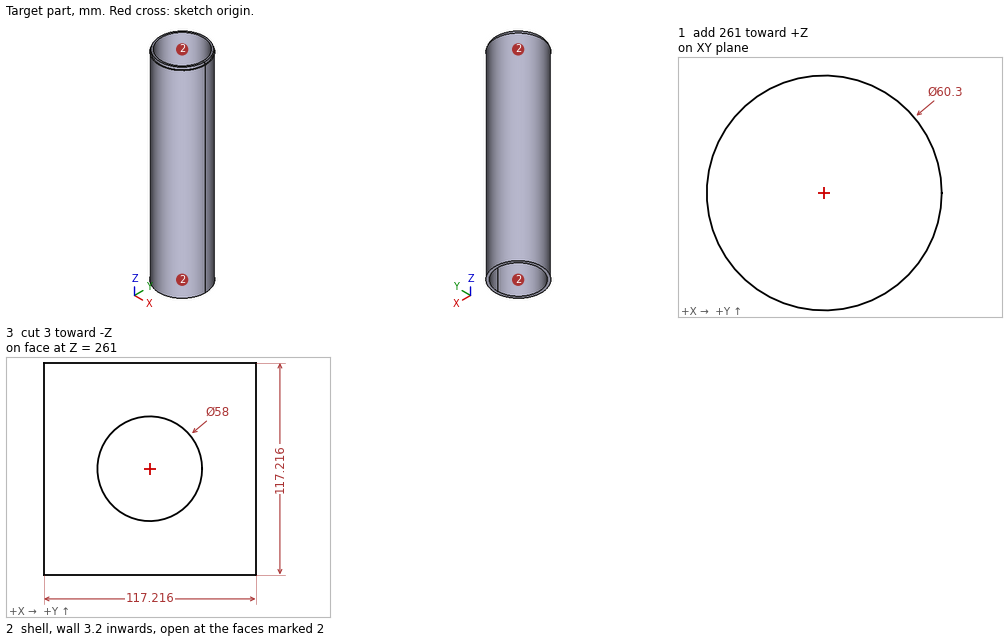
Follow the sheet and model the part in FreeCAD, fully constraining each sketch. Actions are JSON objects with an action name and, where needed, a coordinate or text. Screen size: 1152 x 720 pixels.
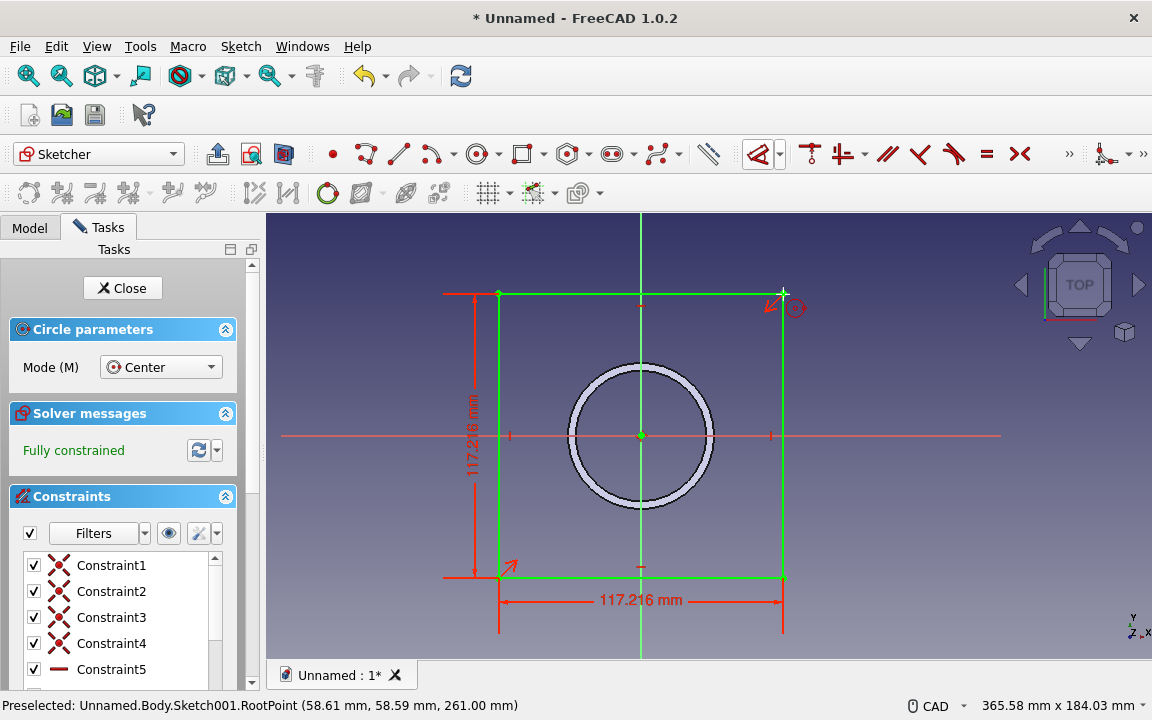
{"action": "left_click", "coordinate": [641, 436]}
{"action": "mouse_move", "coordinate": [691, 386]}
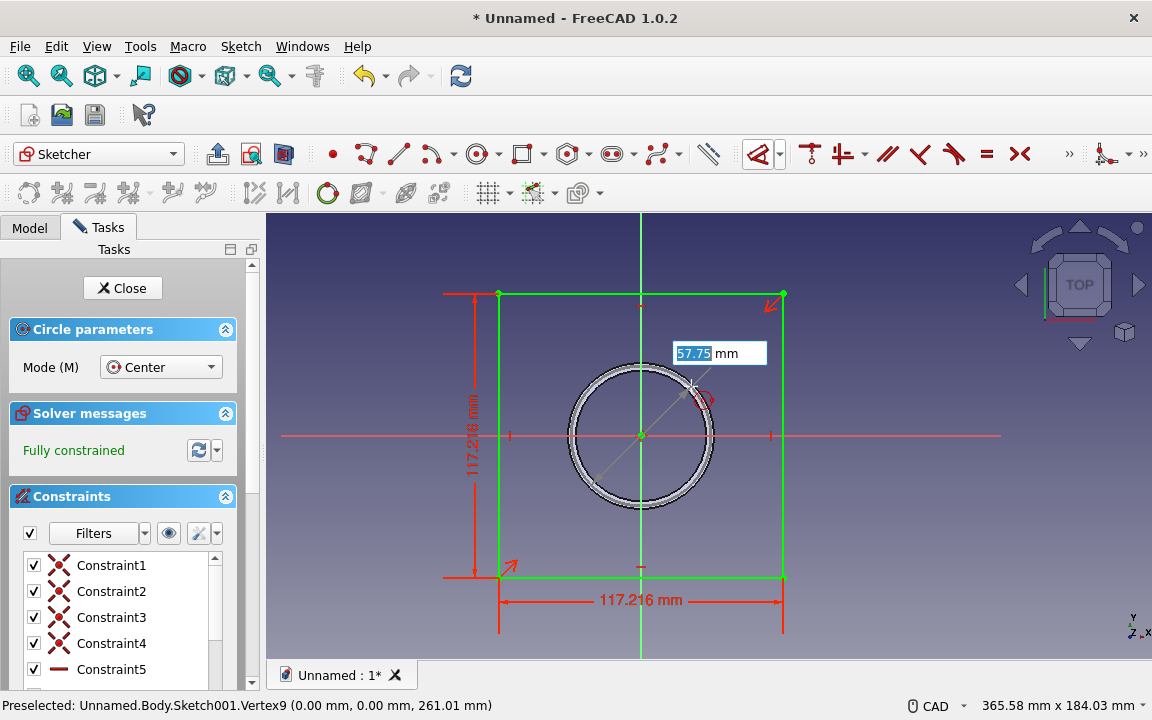
{"action": "type", "text": "58"}
{"action": "key", "text": "Return"}
{"action": "key", "text": "Escape"}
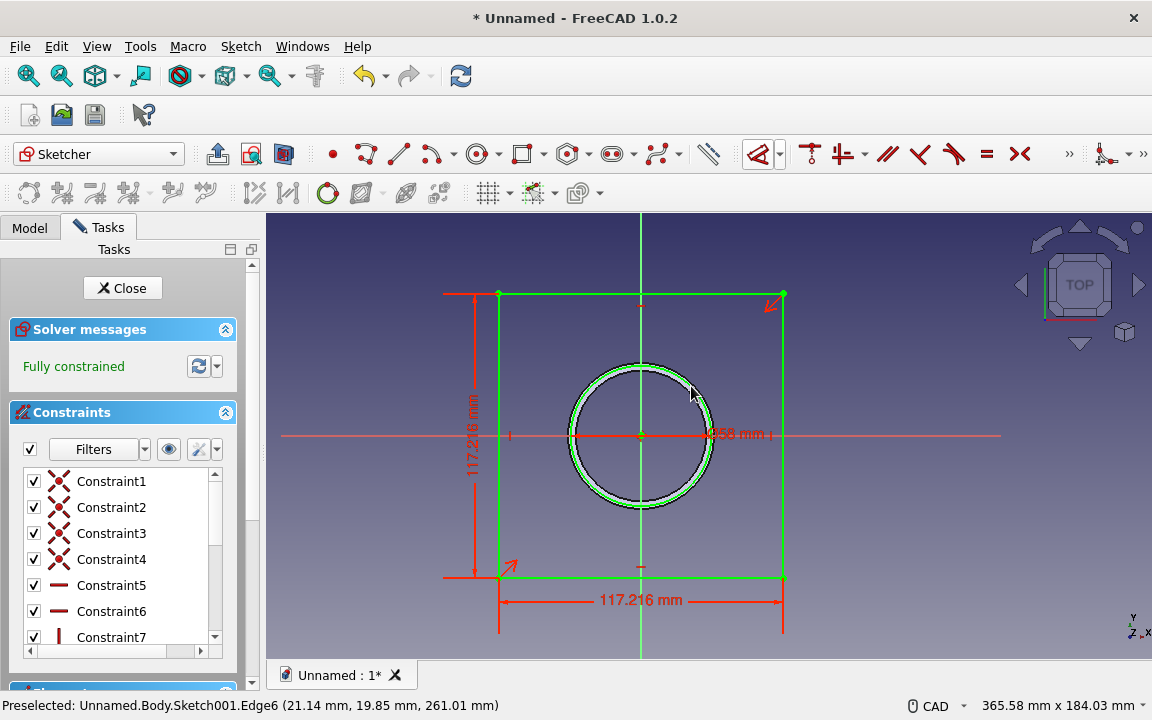
{"action": "left_click", "coordinate": [123, 288]}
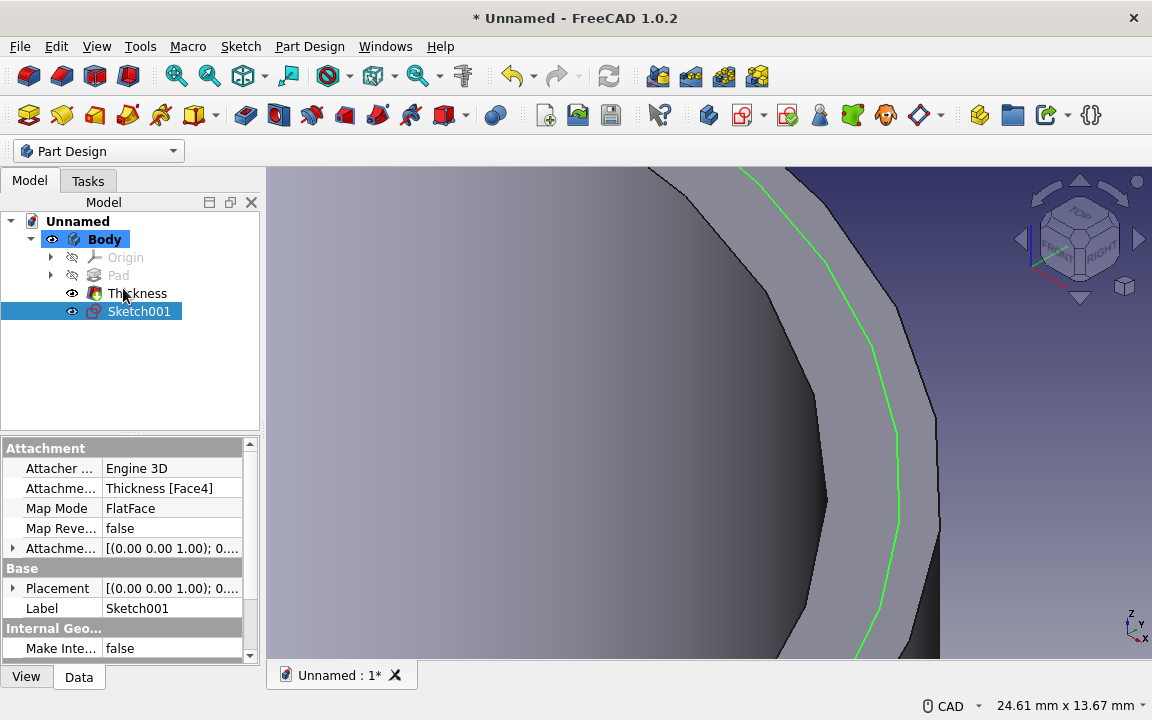
{"action": "left_click", "coordinate": [246, 116]}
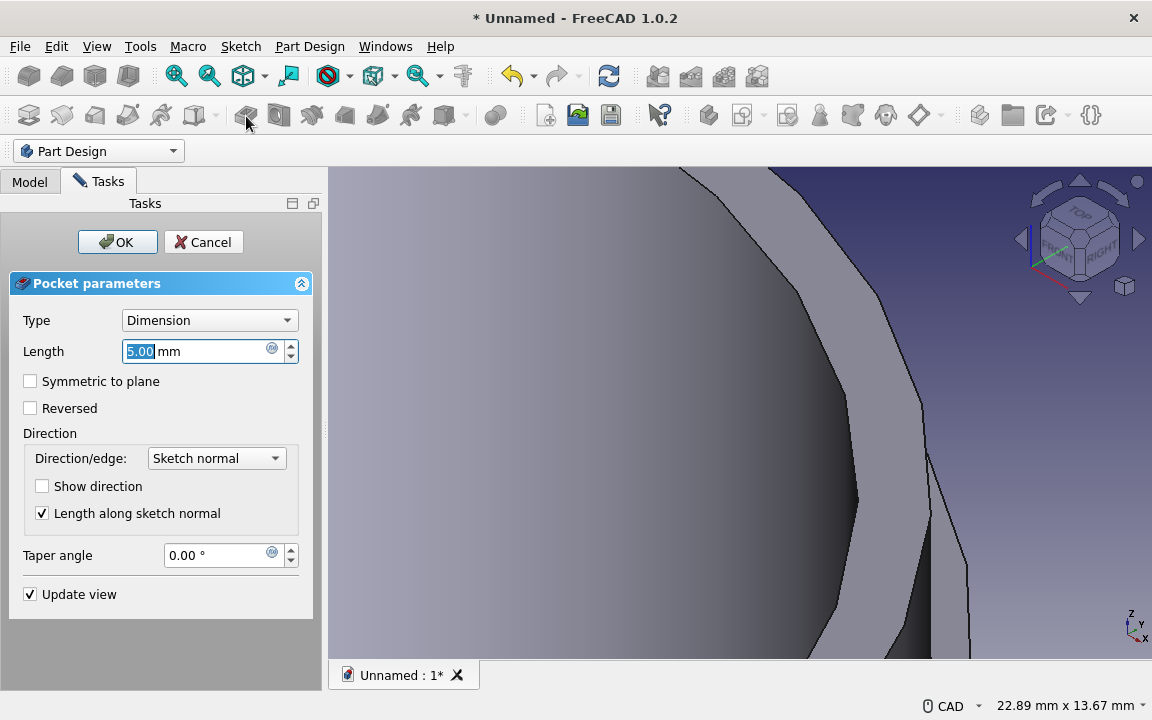
{"action": "type", "text": "3"}
{"action": "key", "text": "Tab"}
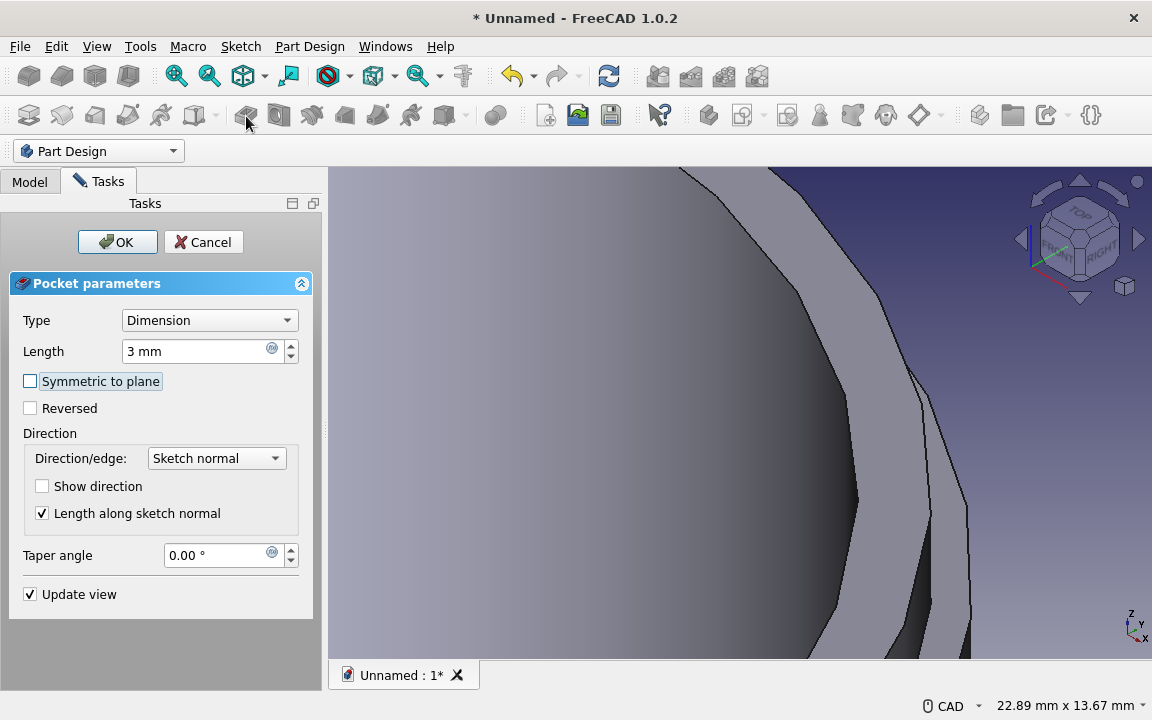
{"action": "left_click", "coordinate": [118, 242]}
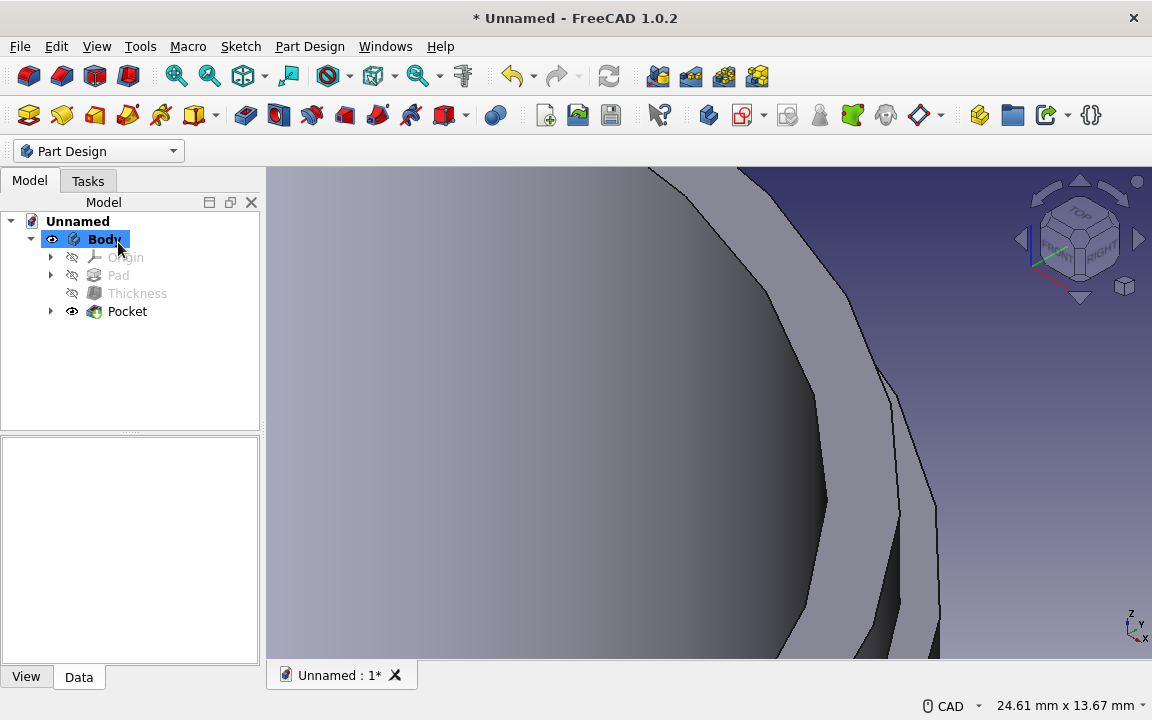
{"action": "key", "text": "v f"}